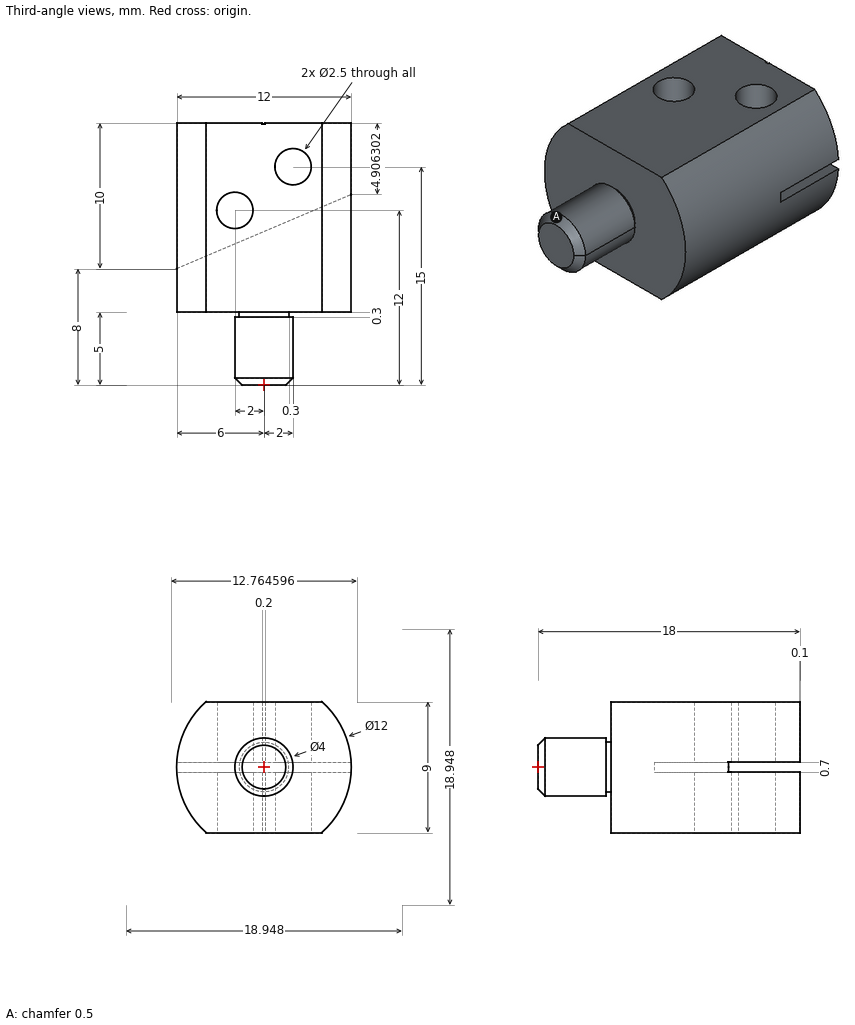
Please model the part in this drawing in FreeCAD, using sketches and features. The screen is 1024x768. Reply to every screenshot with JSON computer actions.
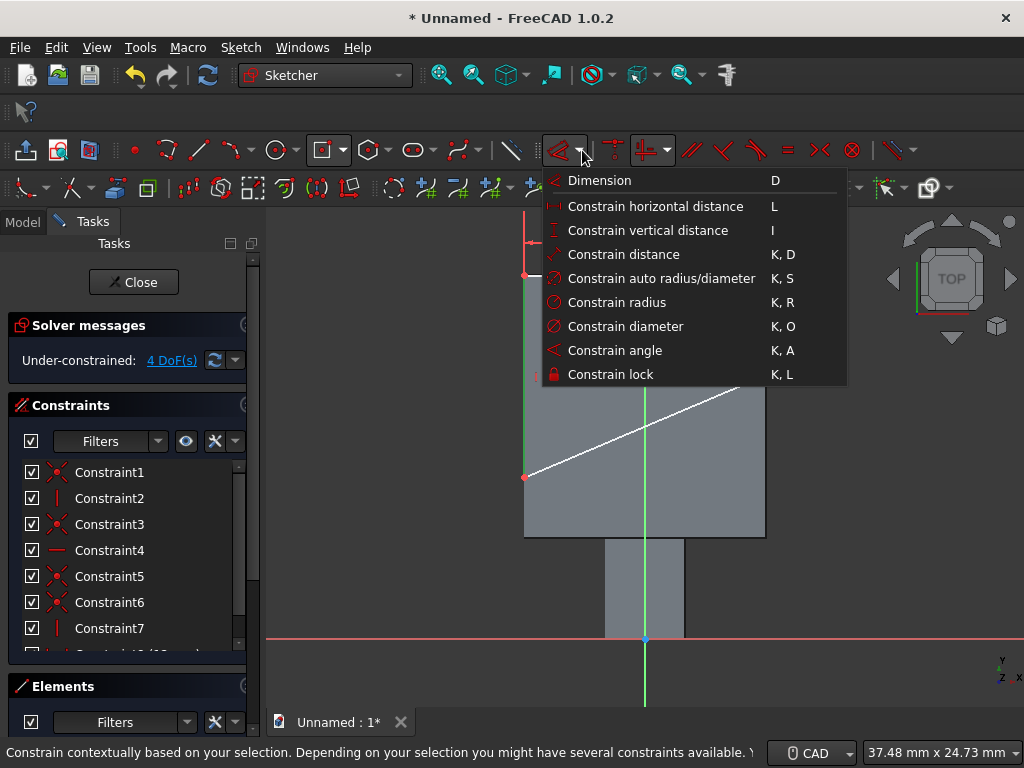
{"action": "left_click", "coordinate": [695, 230]}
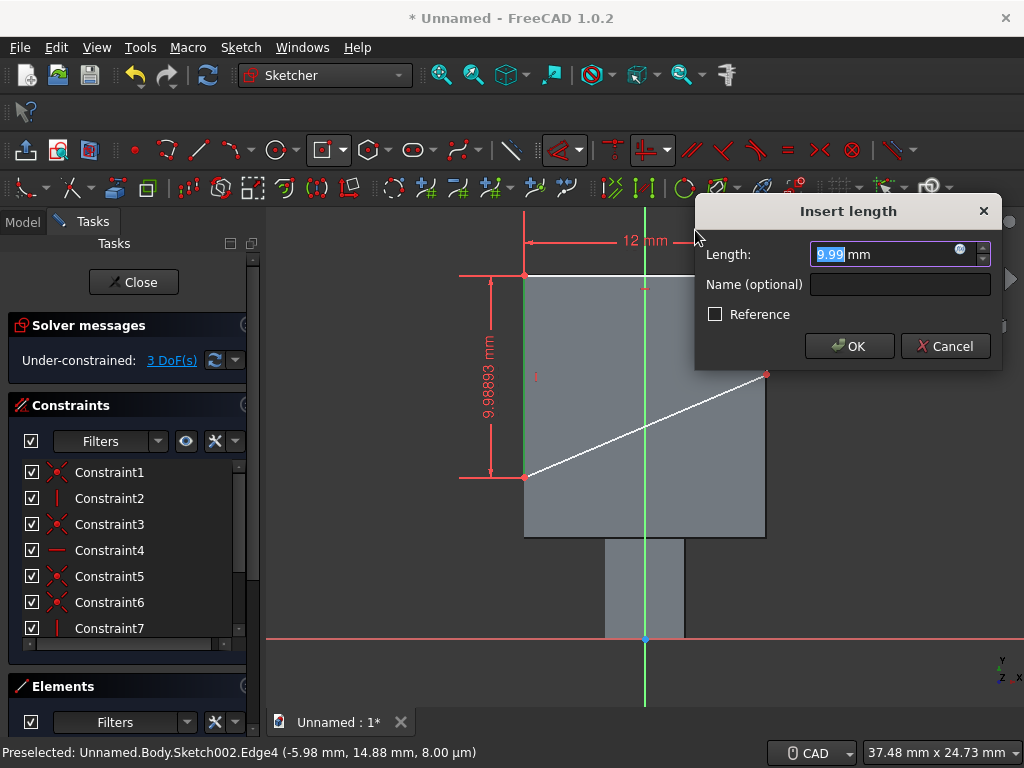
{"action": "type", "text": "10"}
{"action": "key", "text": "Return"}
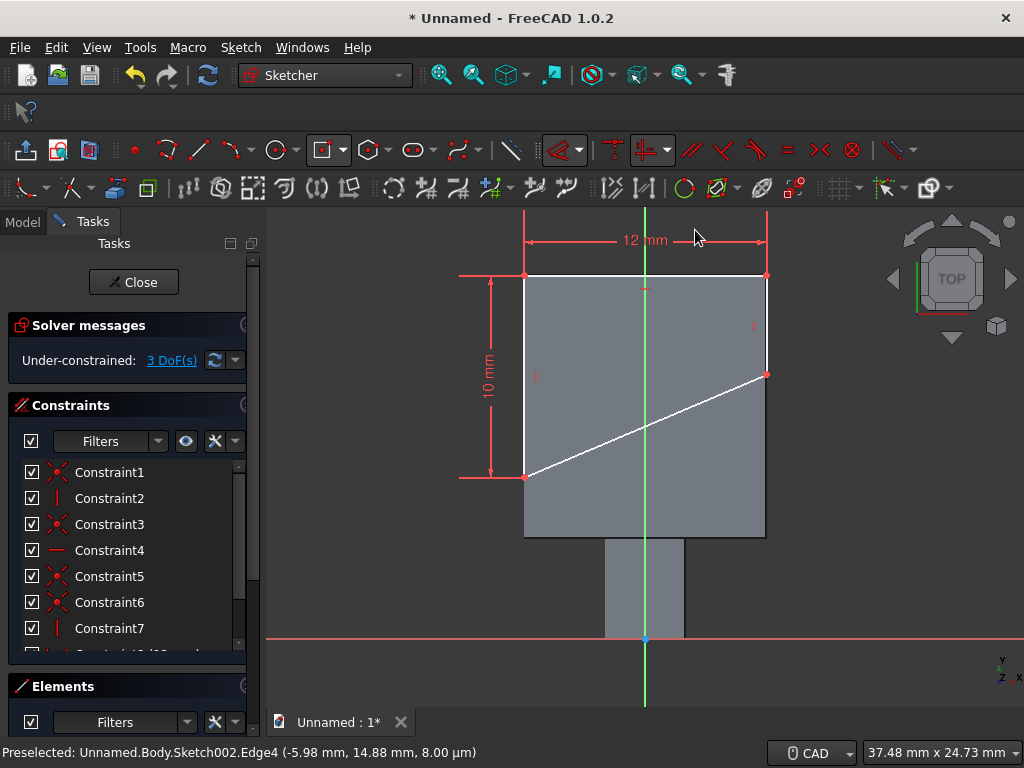
{"action": "left_click", "coordinate": [524, 478]}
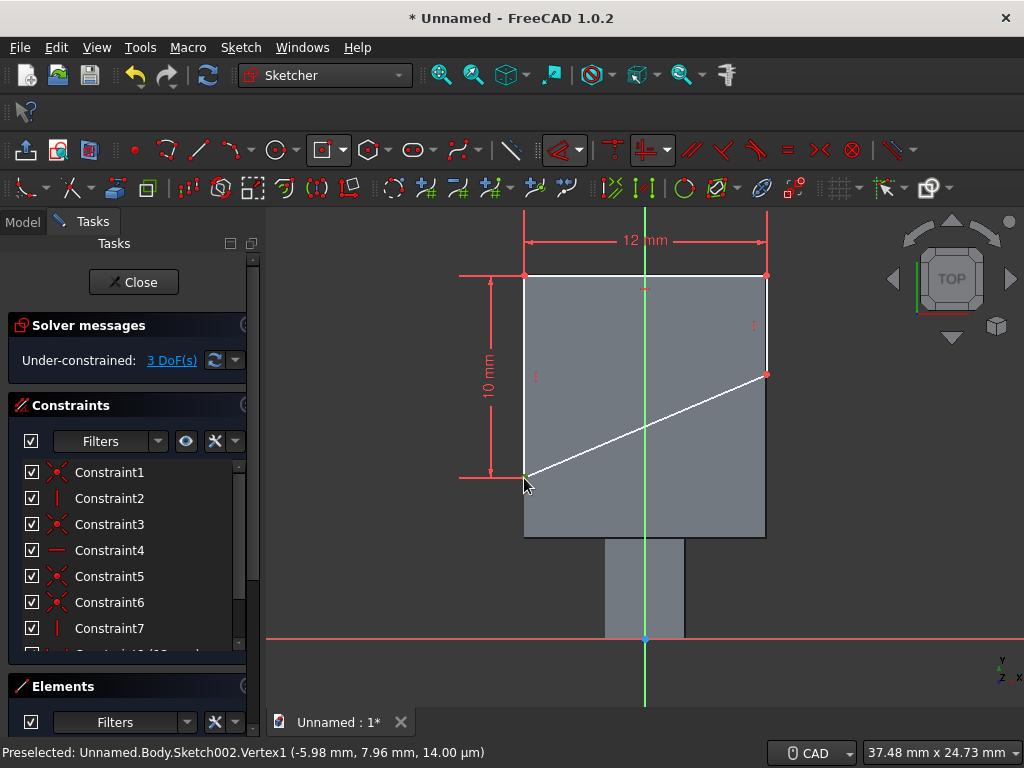
{"action": "left_click", "coordinate": [582, 150]}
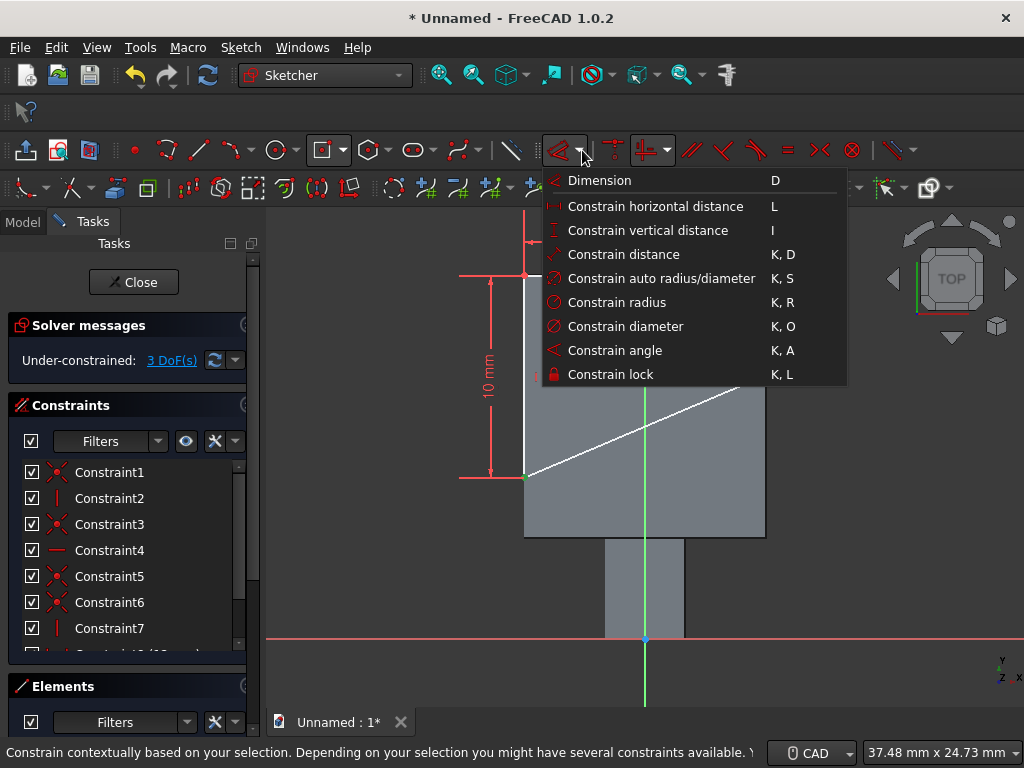
{"action": "left_click", "coordinate": [695, 206]}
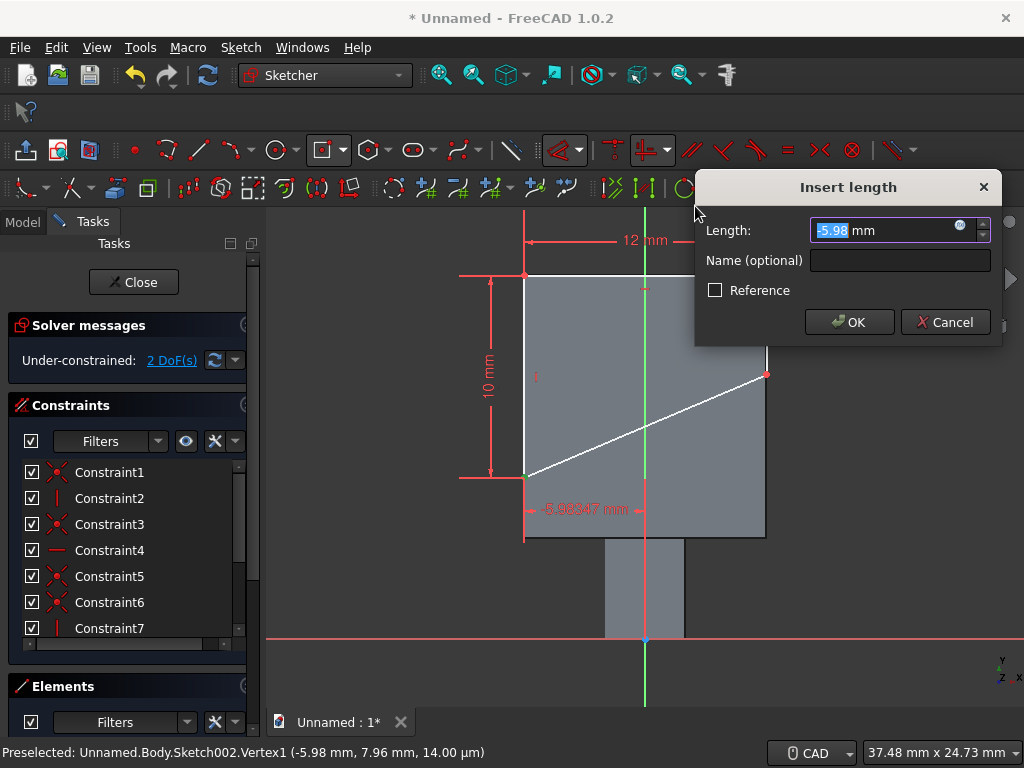
{"action": "type", "text": "-6"}
{"action": "key", "text": "Return"}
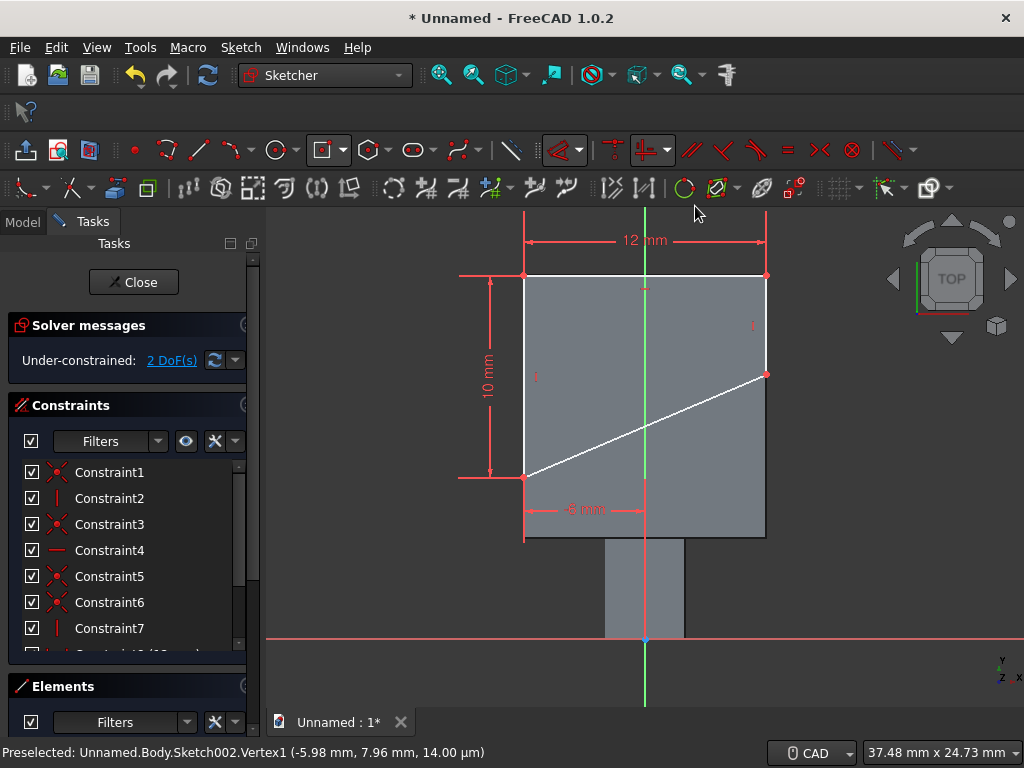
{"action": "left_click", "coordinate": [524, 478]}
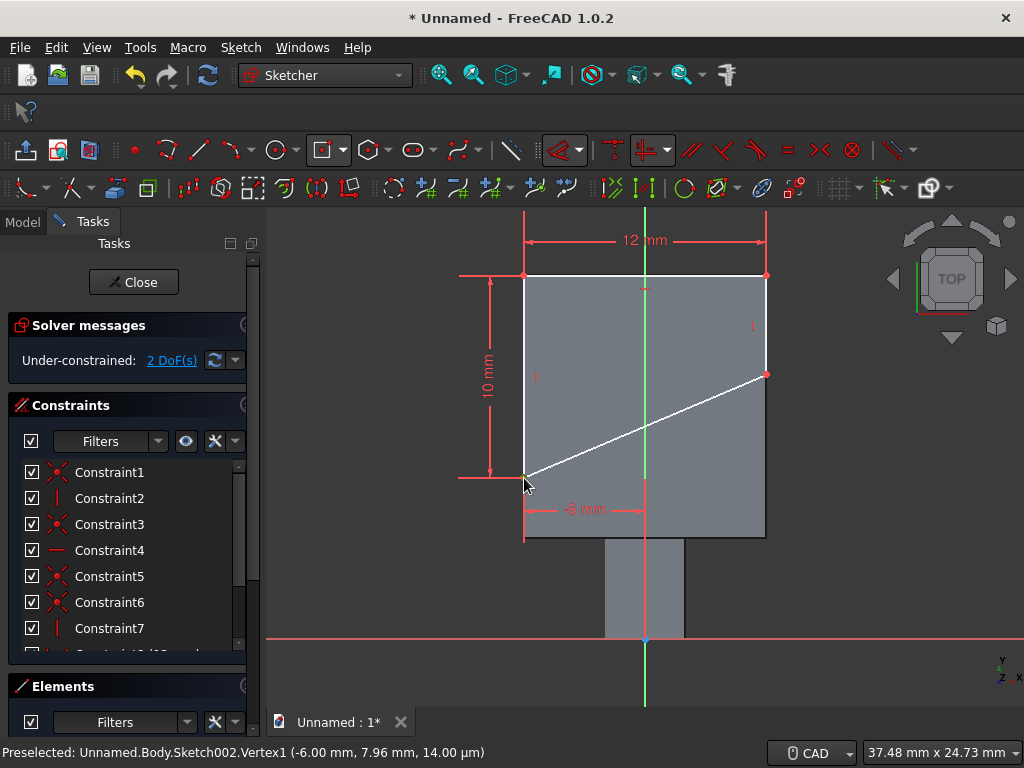
{"action": "left_click", "coordinate": [582, 150]}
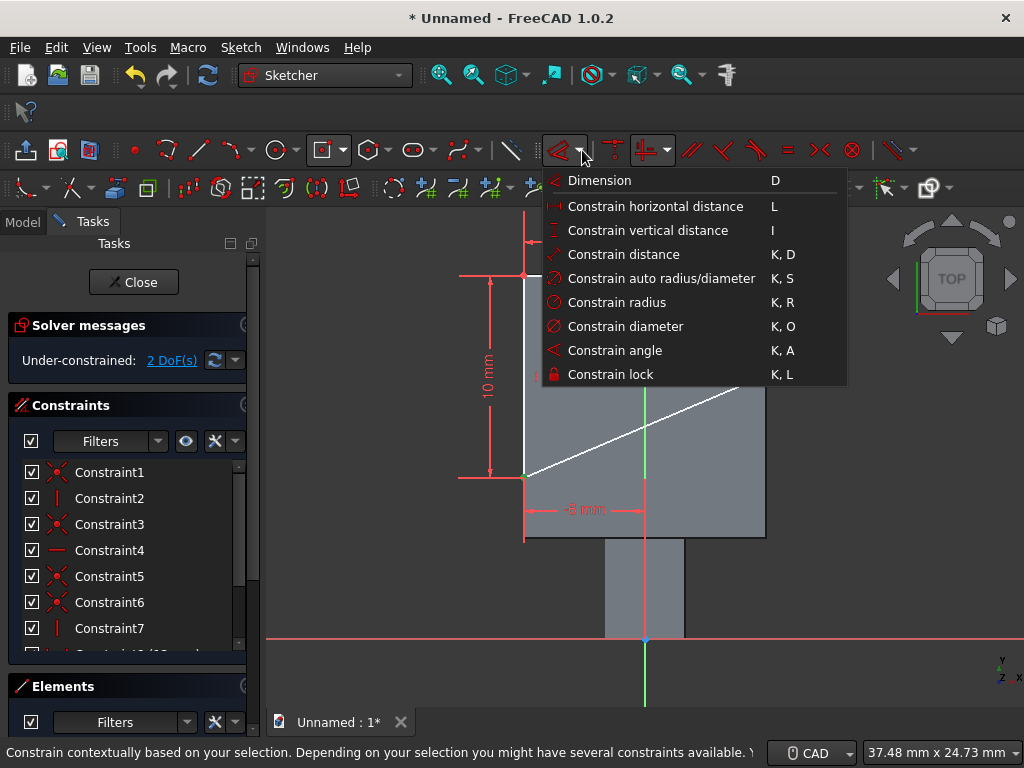
{"action": "left_click", "coordinate": [695, 230]}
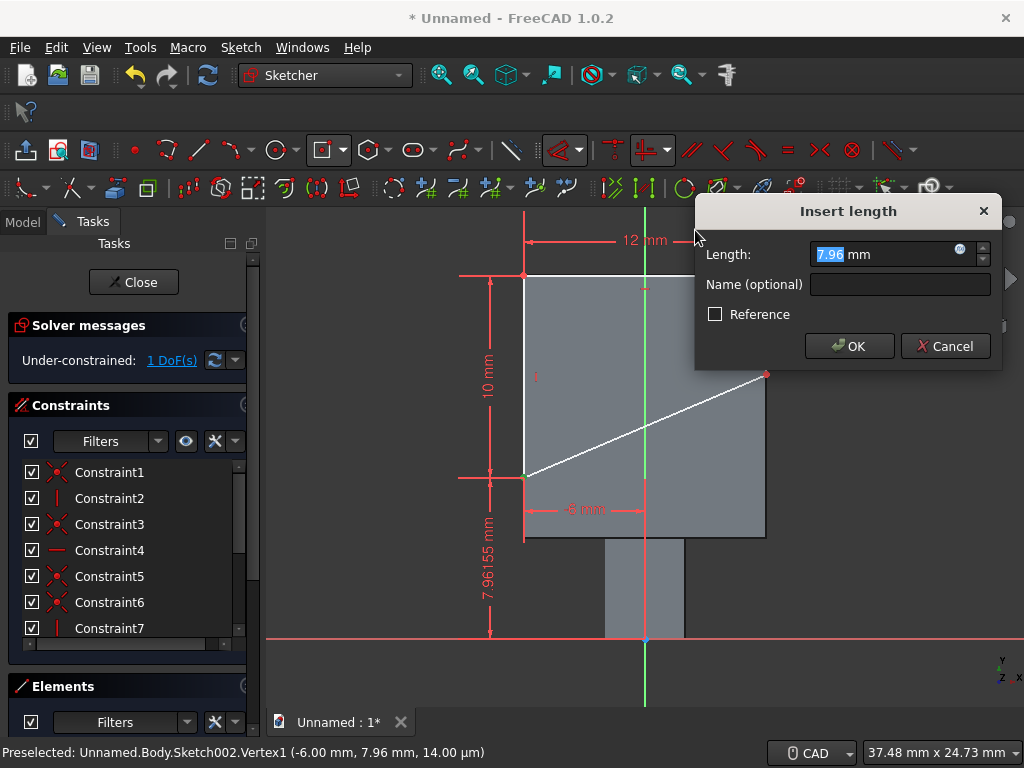
{"action": "type", "text": "8"}
{"action": "key", "text": "Return"}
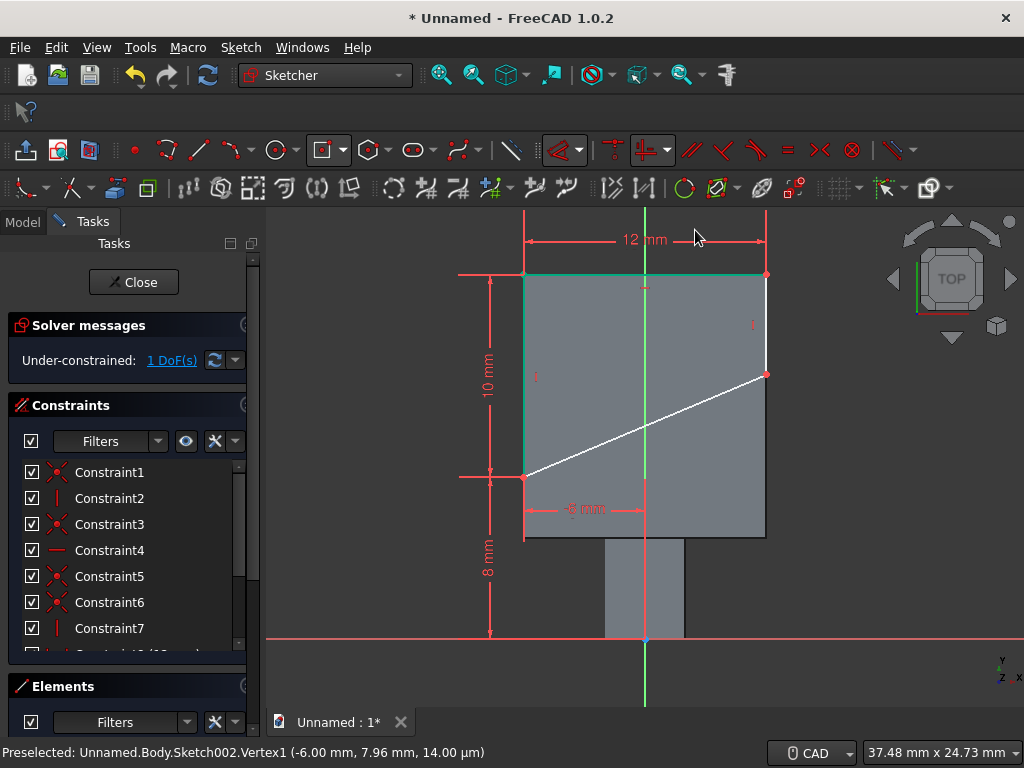
{"action": "left_click", "coordinate": [766, 345]}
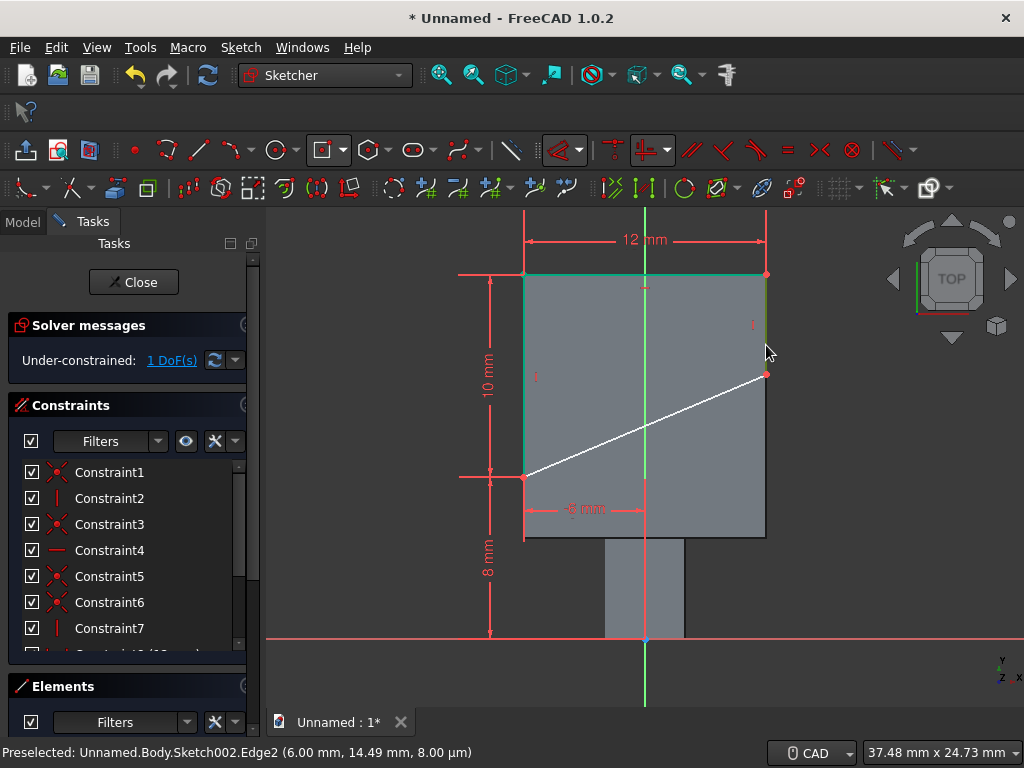
{"action": "left_click", "coordinate": [582, 150]}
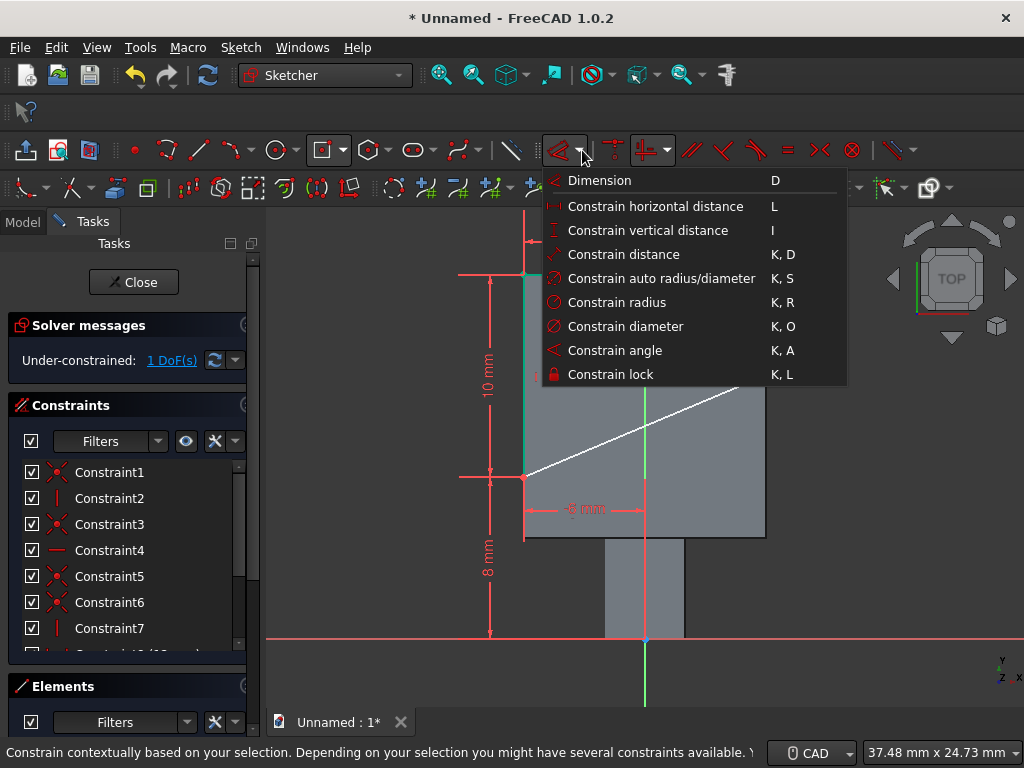
{"action": "left_click", "coordinate": [695, 230]}